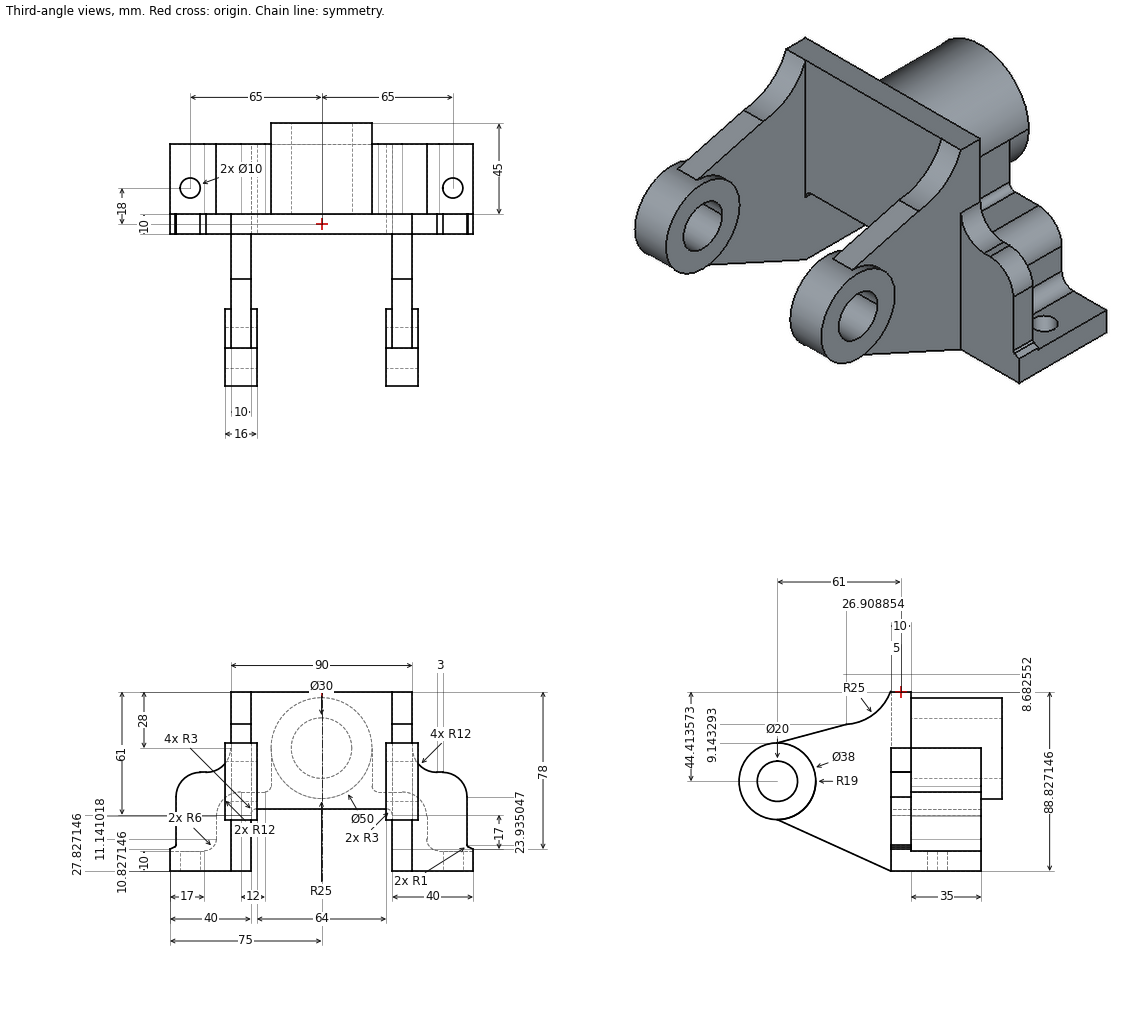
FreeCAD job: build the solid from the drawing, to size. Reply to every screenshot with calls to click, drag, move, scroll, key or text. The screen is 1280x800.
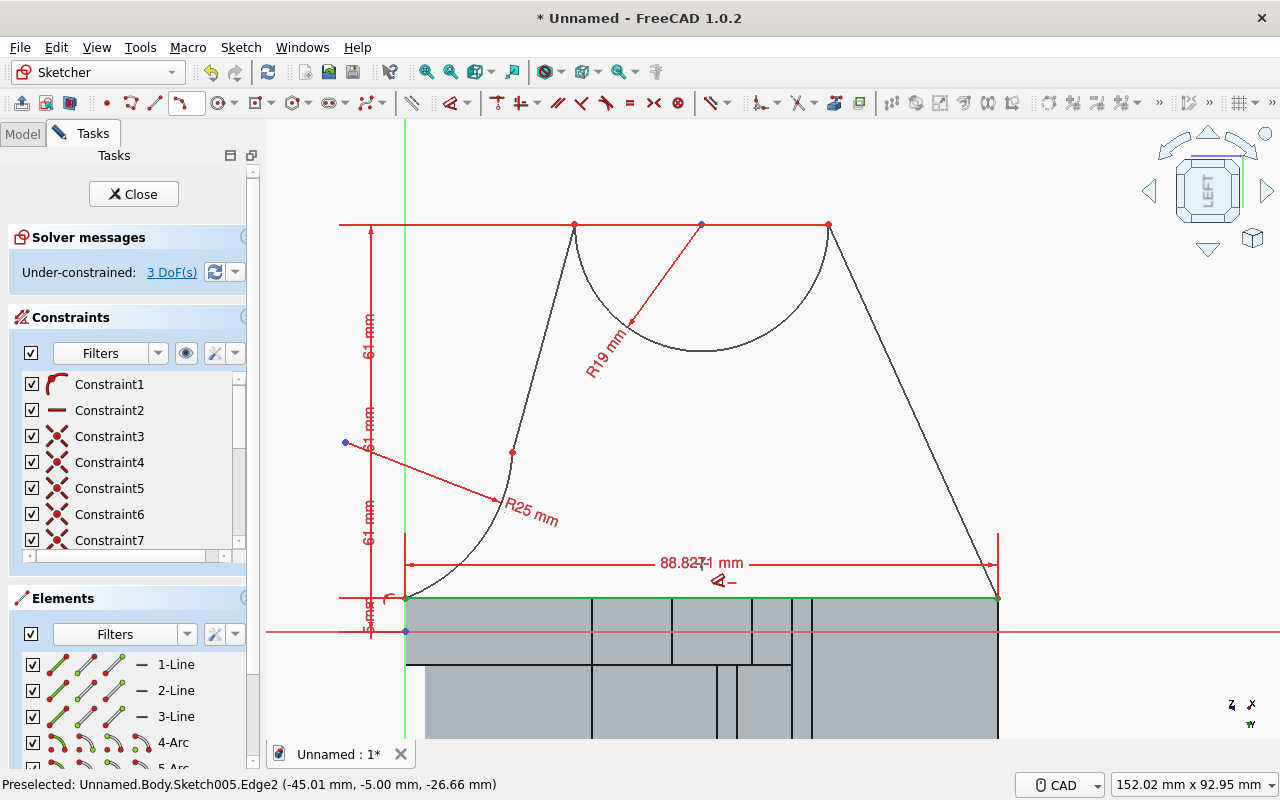
click(556, 293)
click(544, 191)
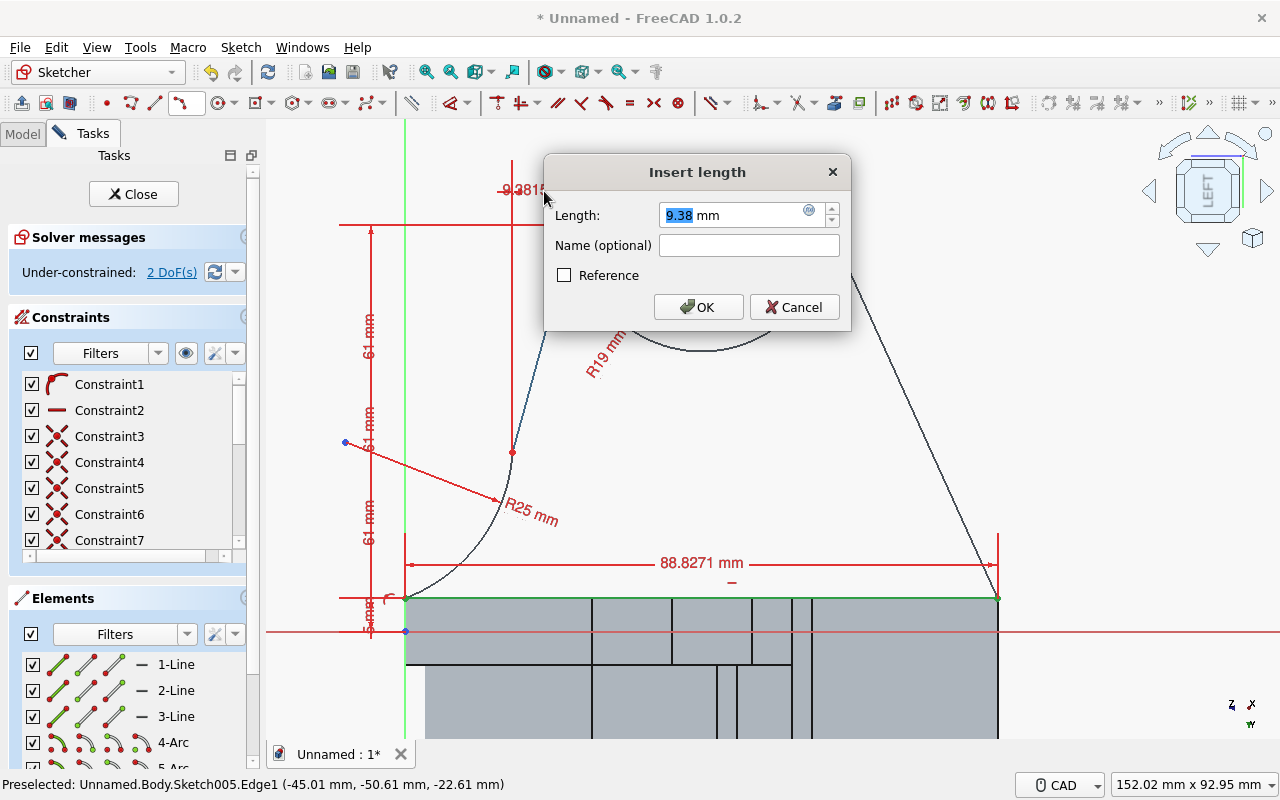
text(9.143293)
key(Return)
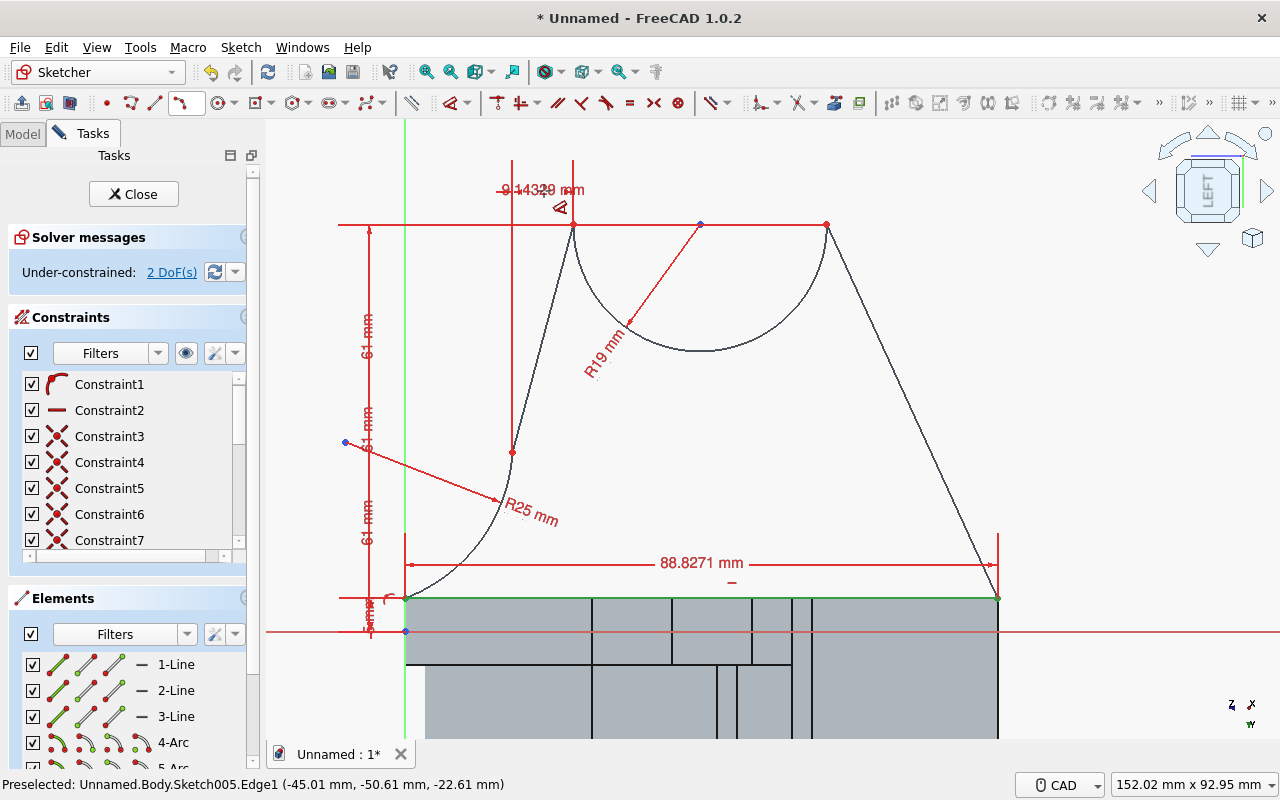
click(346, 442)
click(376, 666)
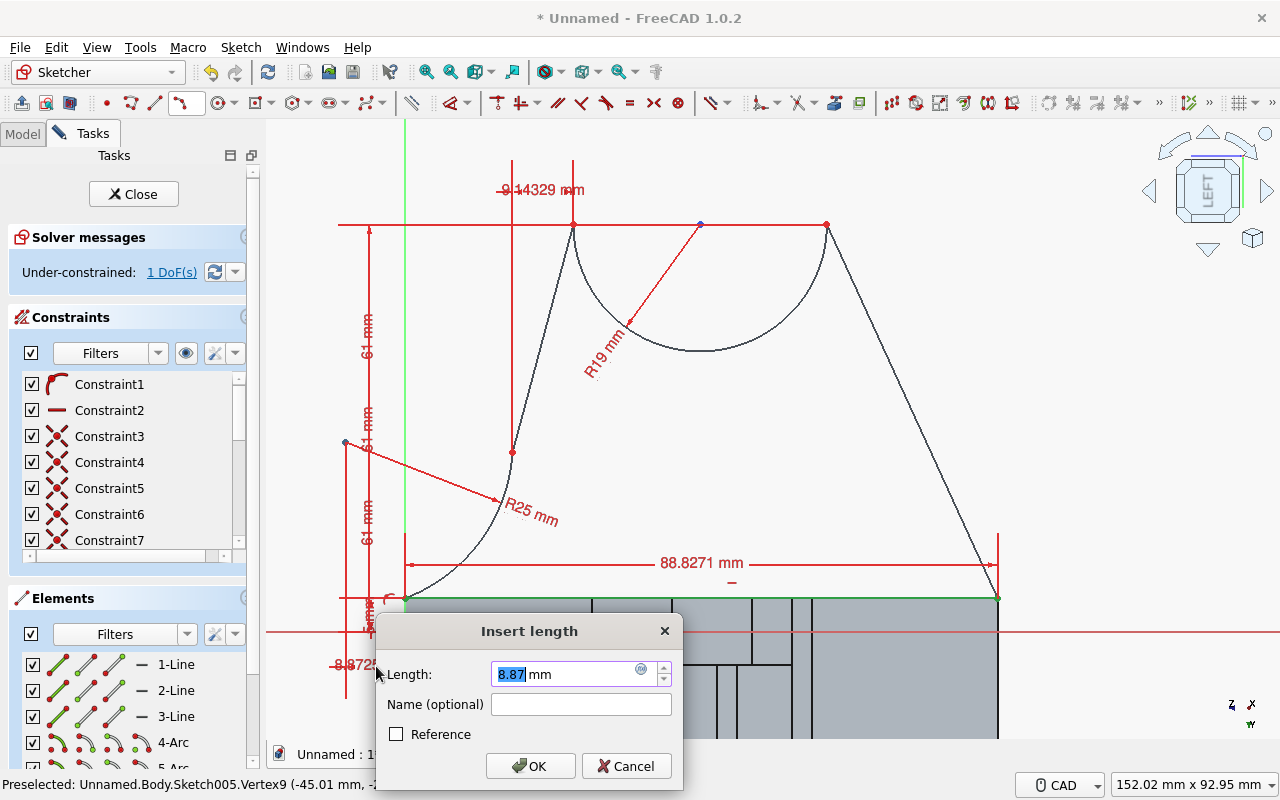
text(8.682552)
key(Return)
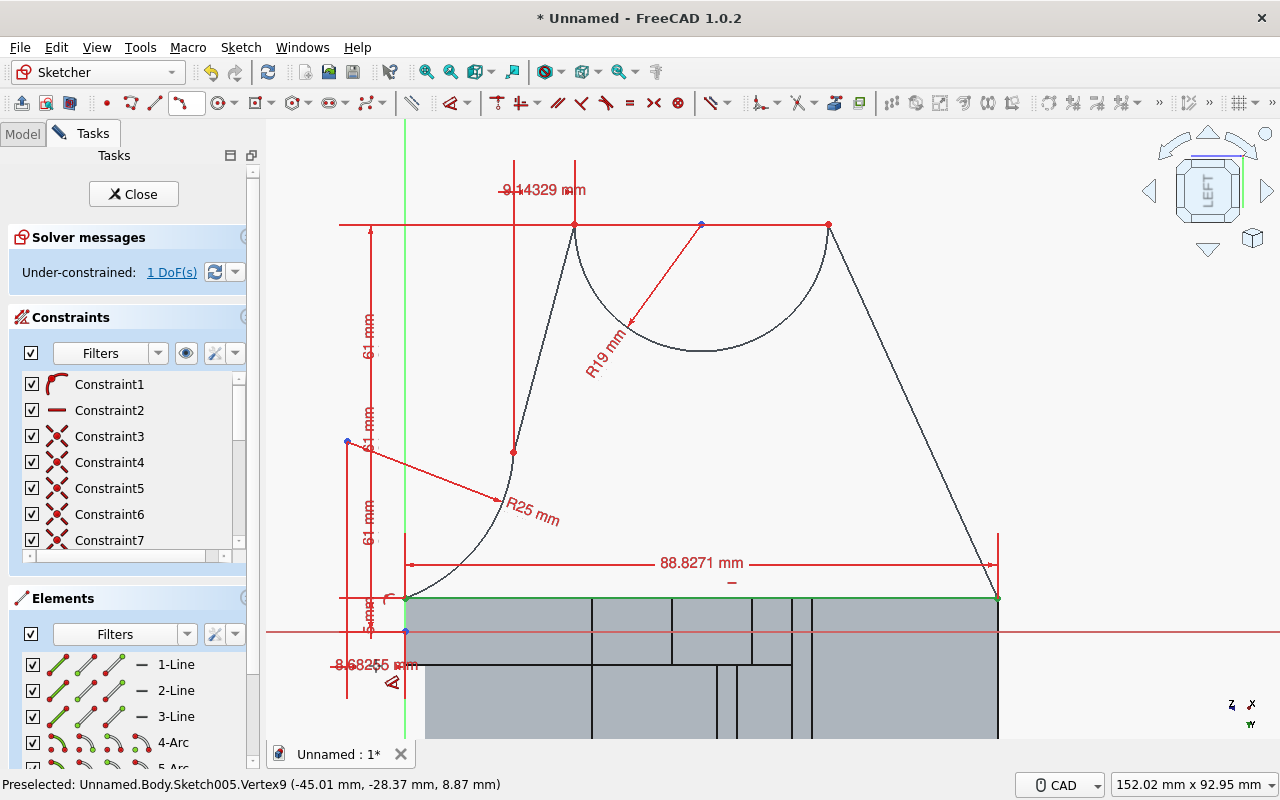
click(514, 453)
click(371, 542)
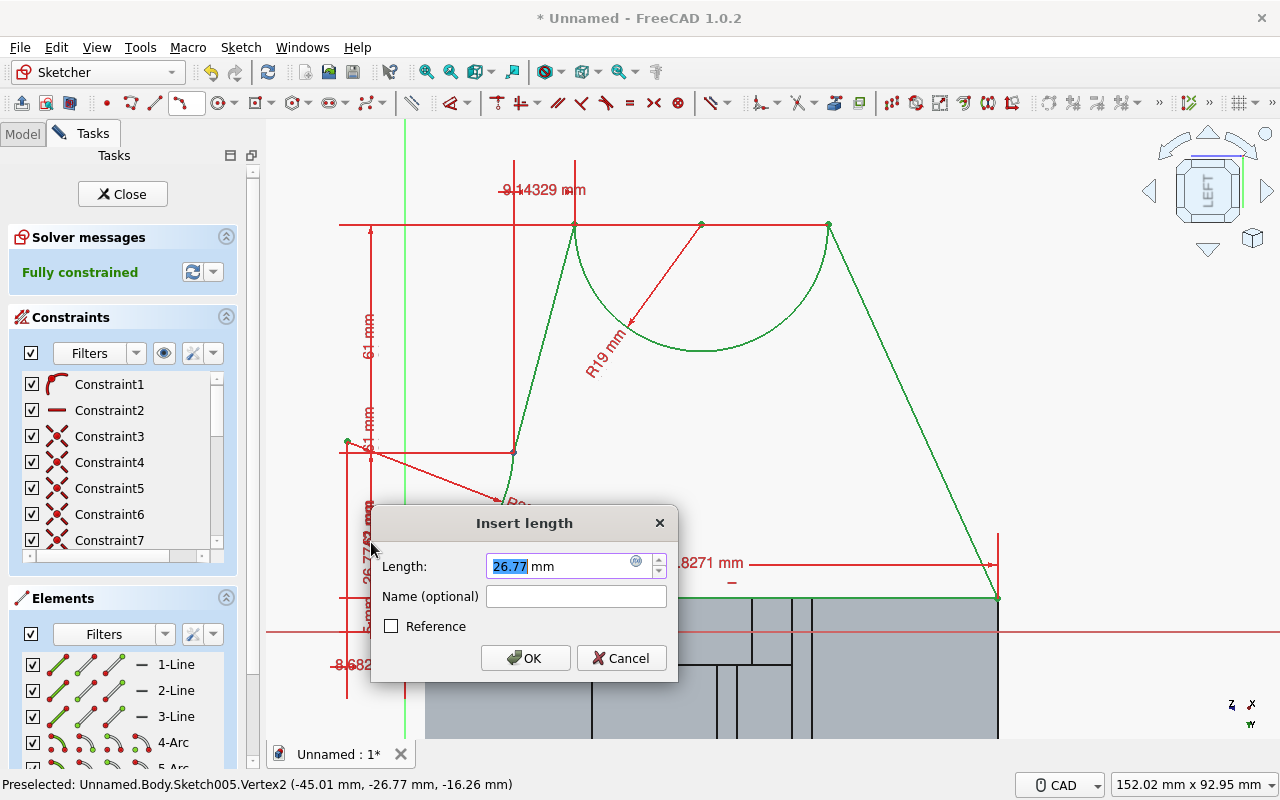
text(26.908854)
key(Return)
key(Escape)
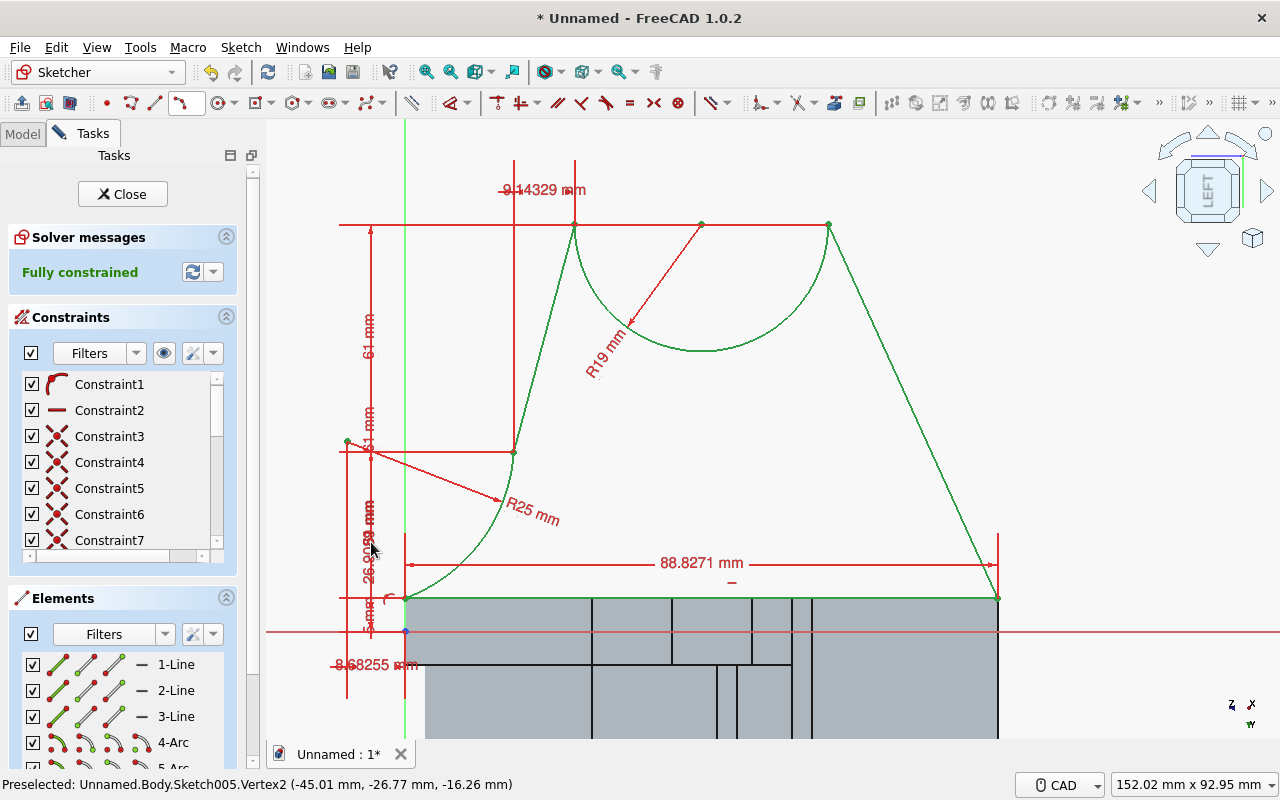
click(123, 194)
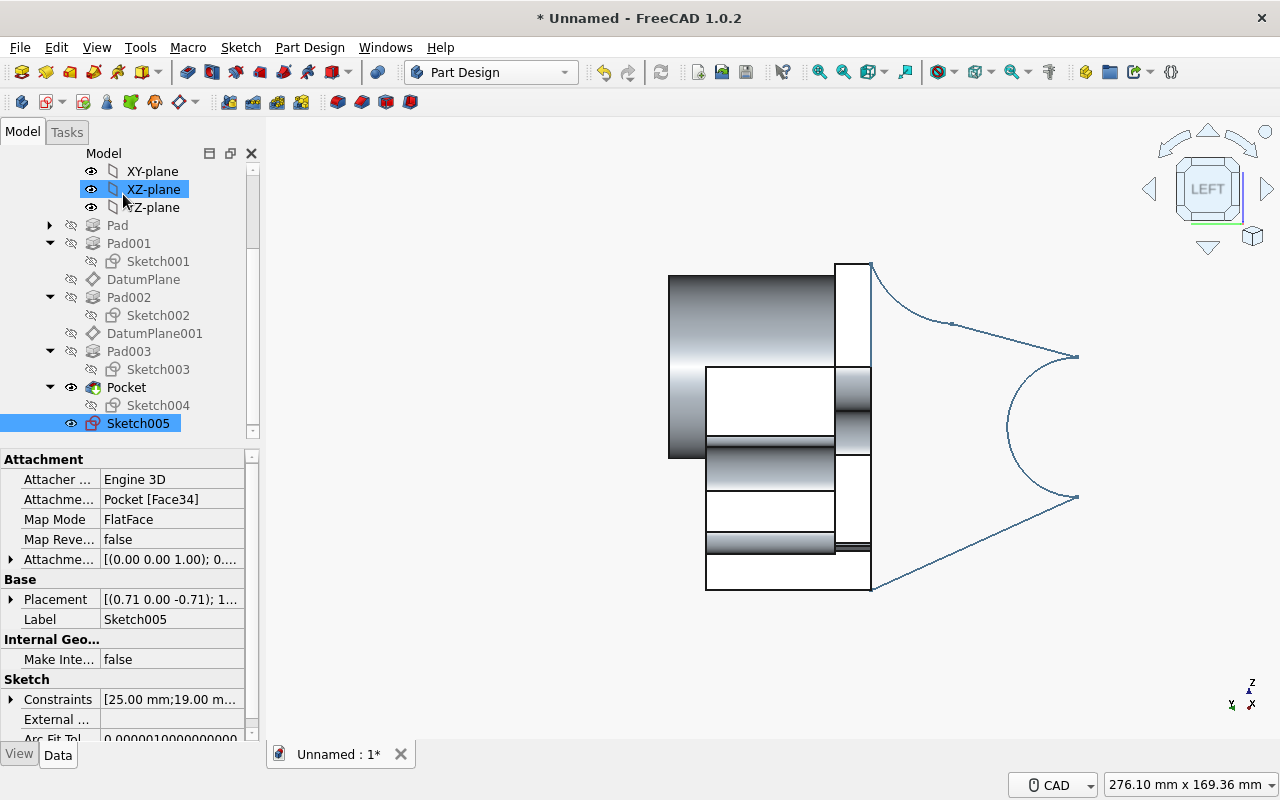
click(22, 72)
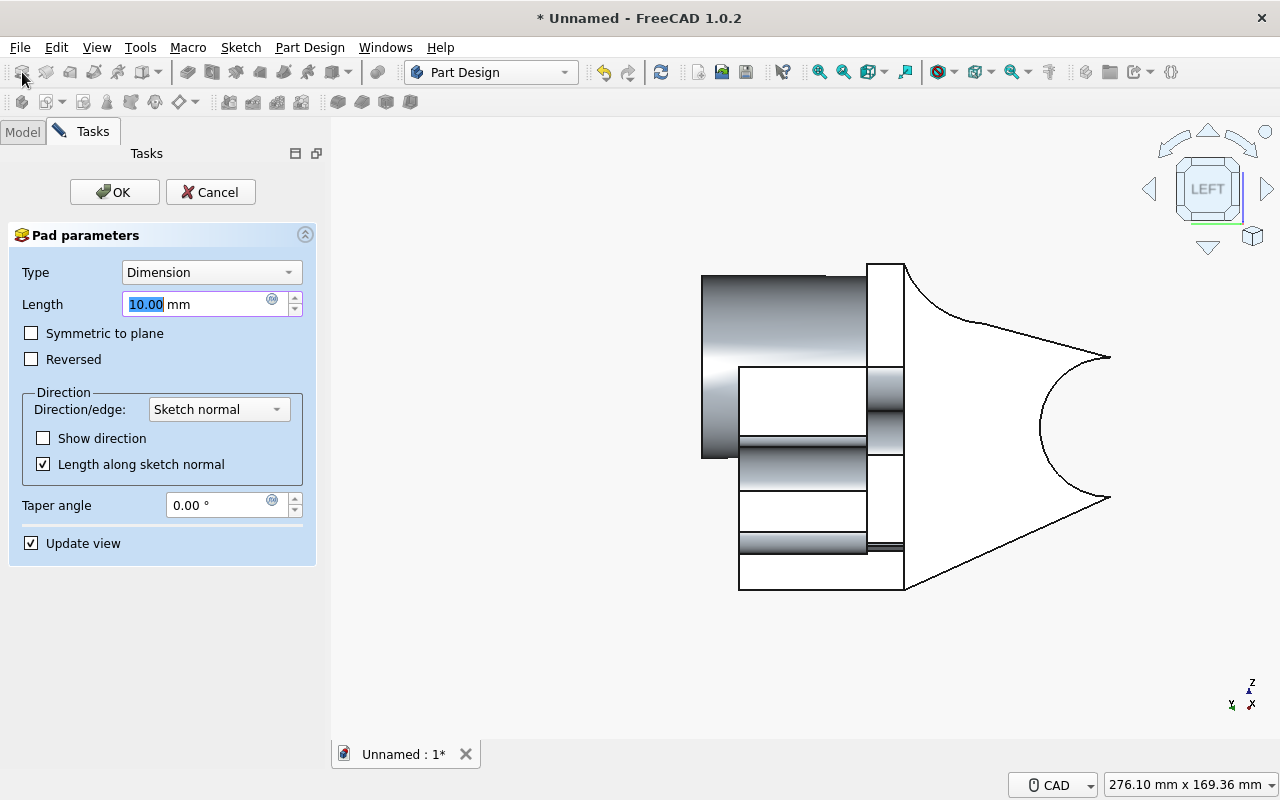
text(10)
key(Tab)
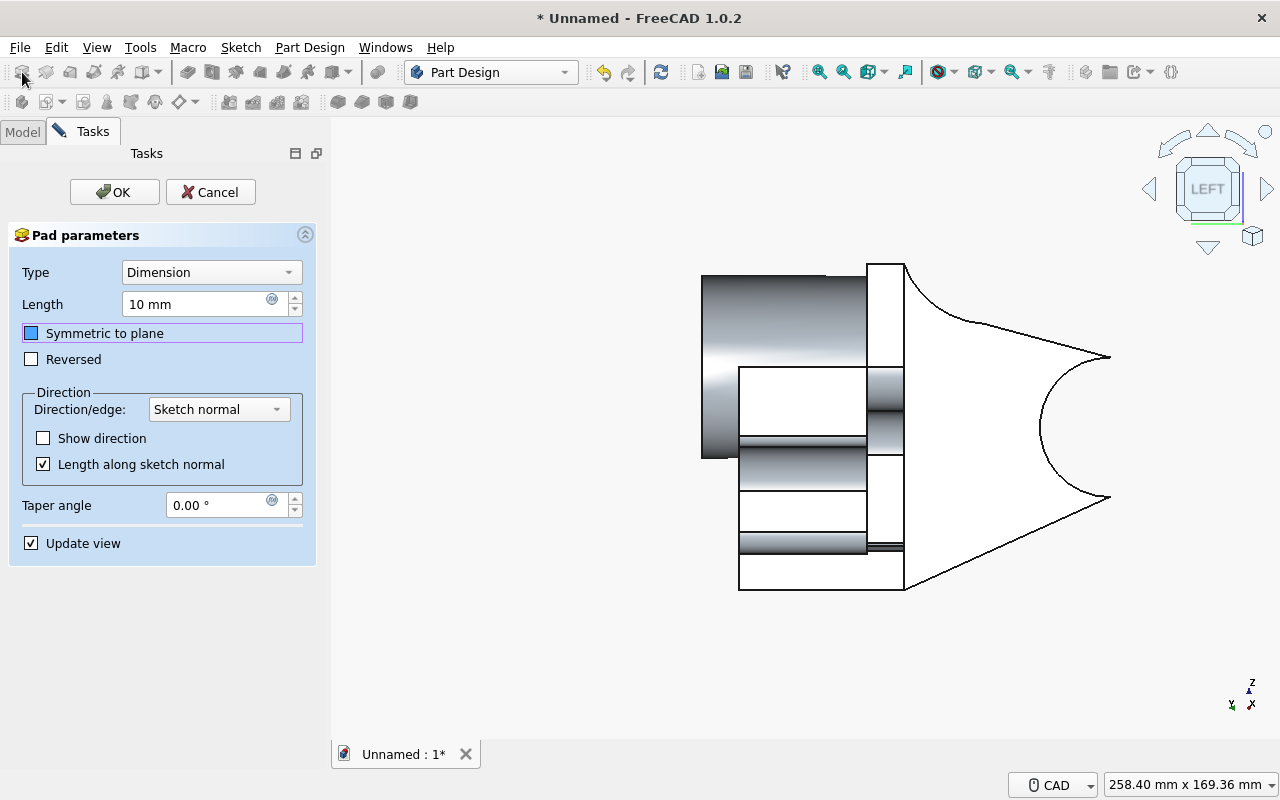
click(30, 359)